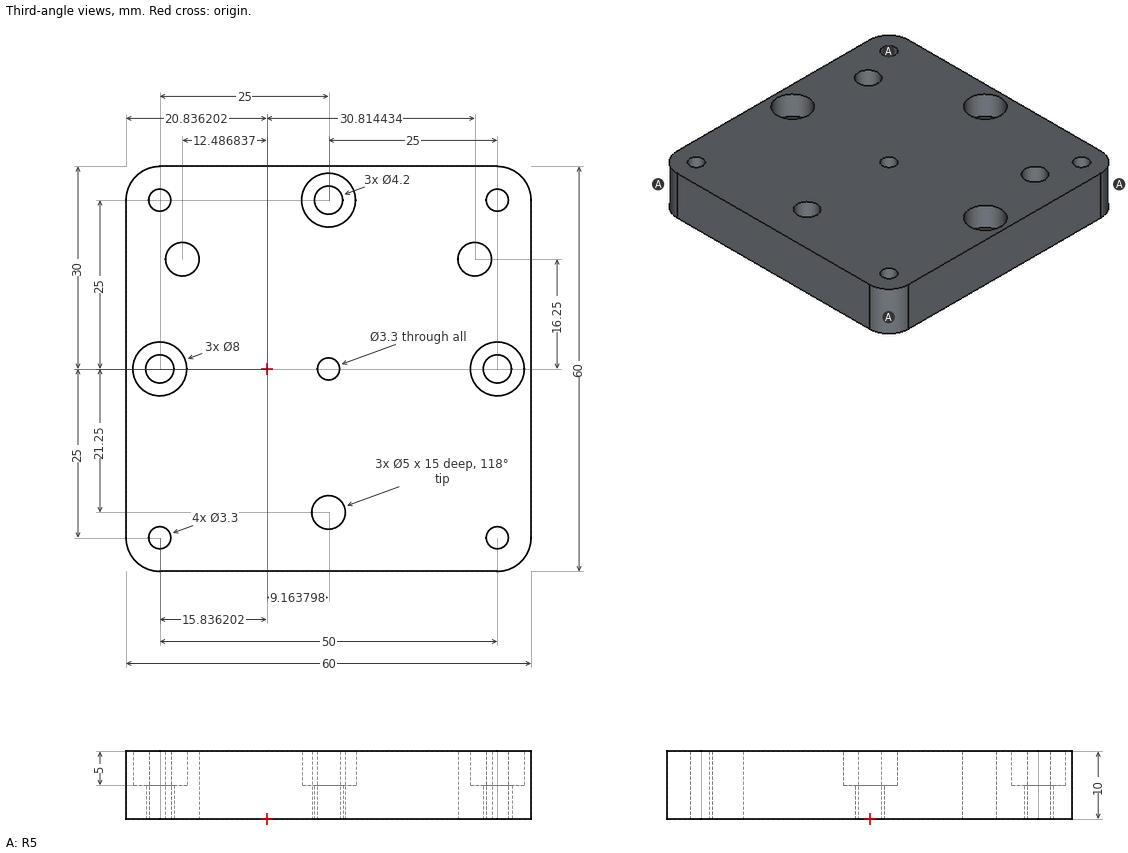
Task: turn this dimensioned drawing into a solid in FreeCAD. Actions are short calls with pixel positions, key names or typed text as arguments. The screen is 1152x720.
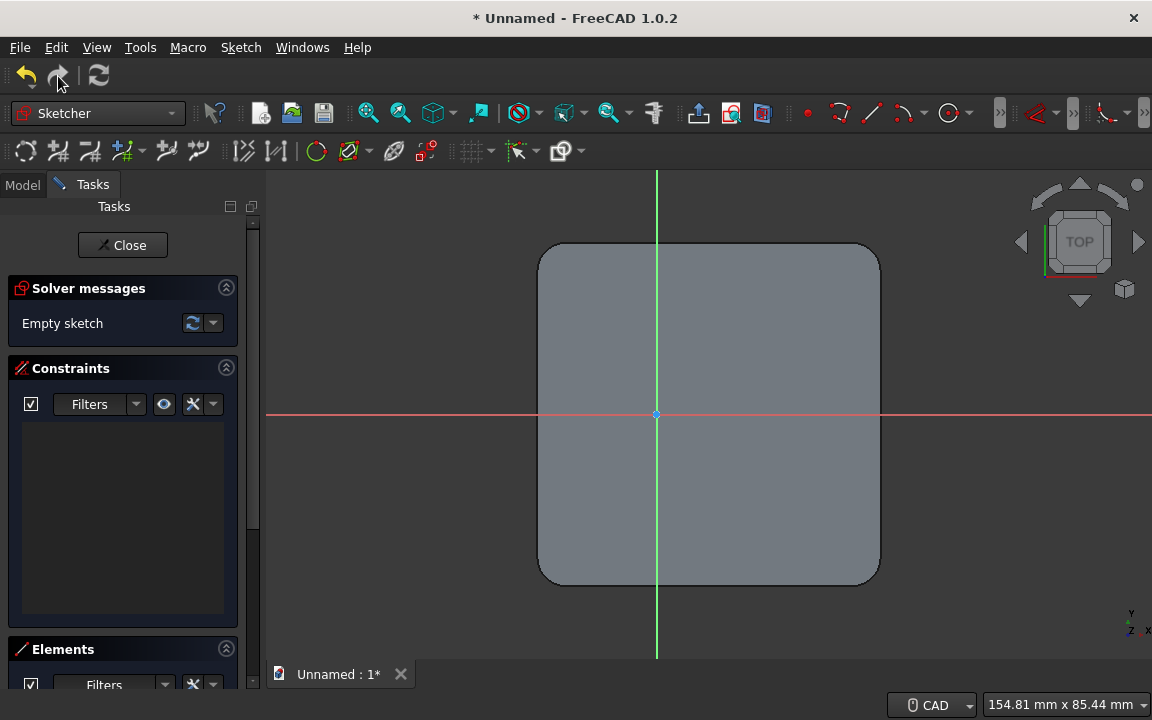
click(950, 114)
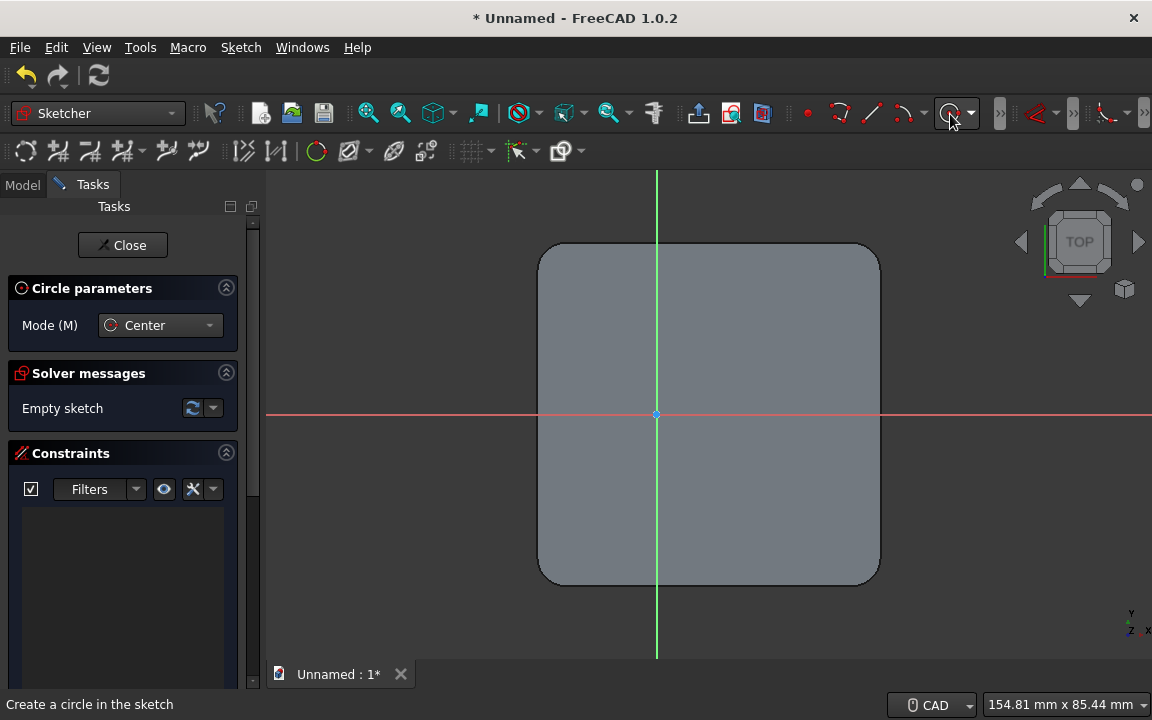
scroll(709, 536, up, 3)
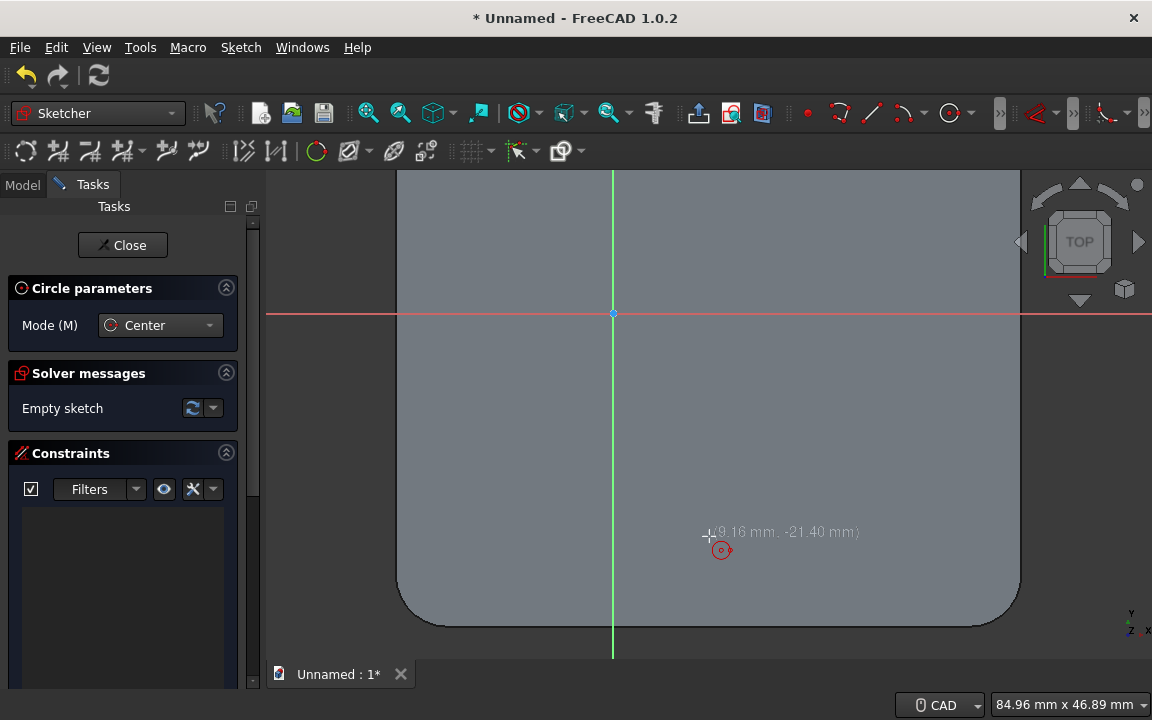
click(709, 536)
move(727, 517)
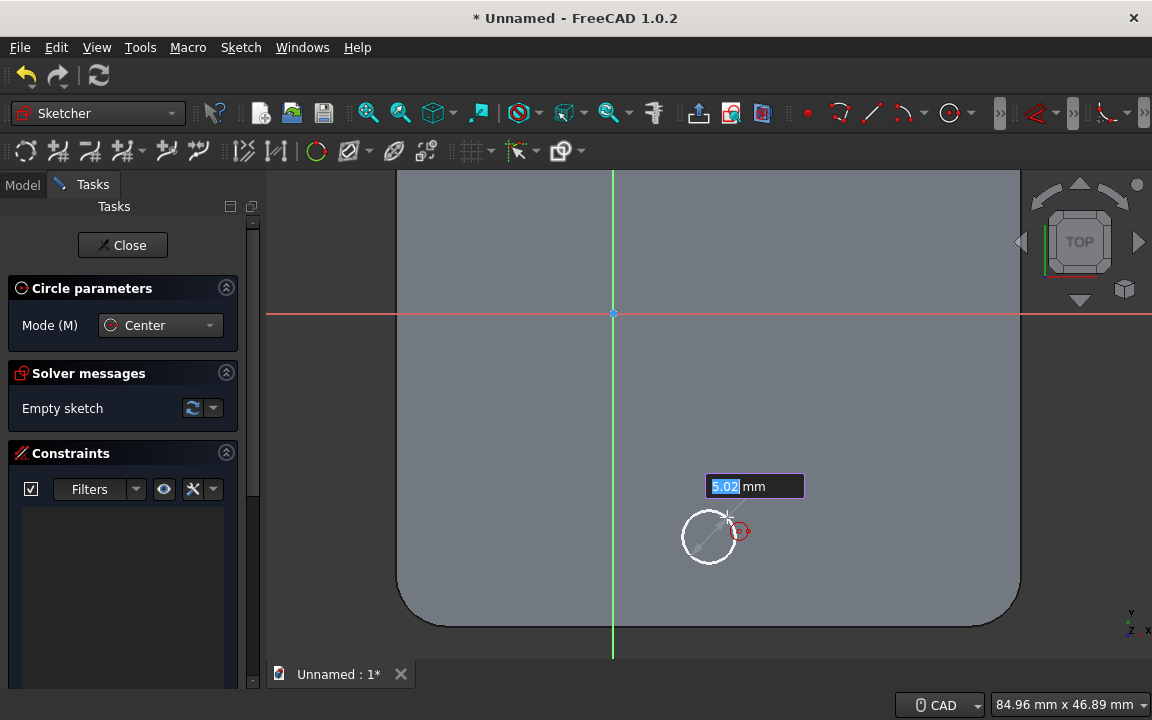
text(5)
key(Return)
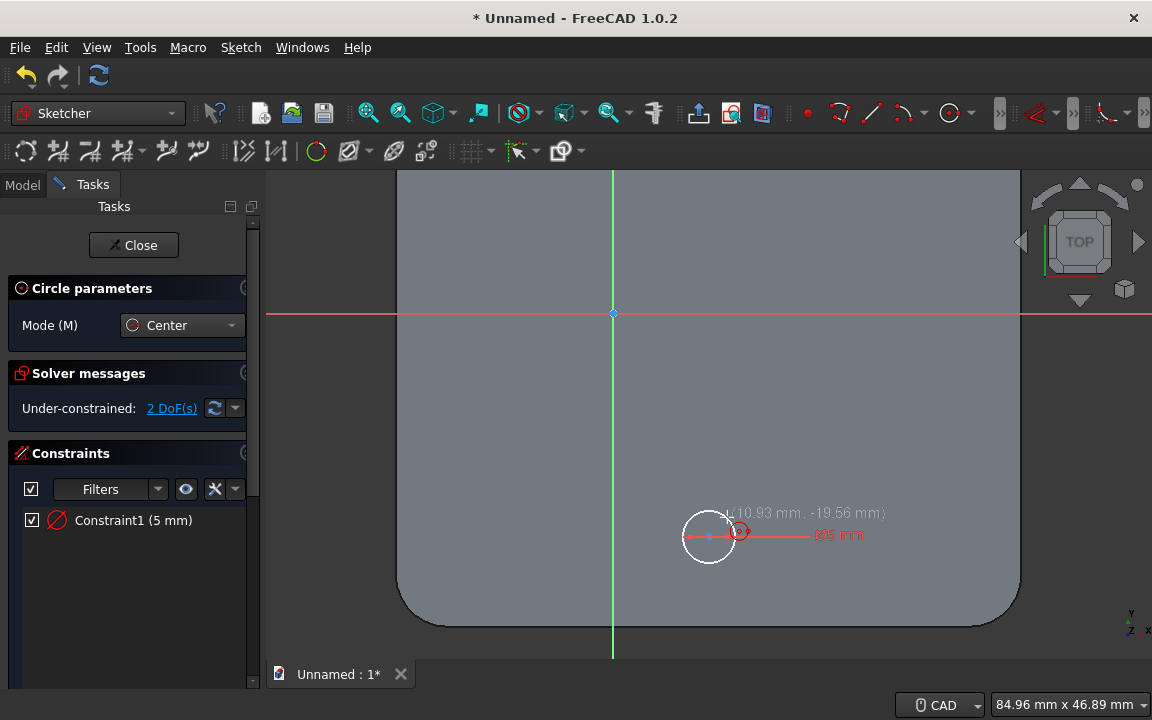
scroll(502, 566, down, 2)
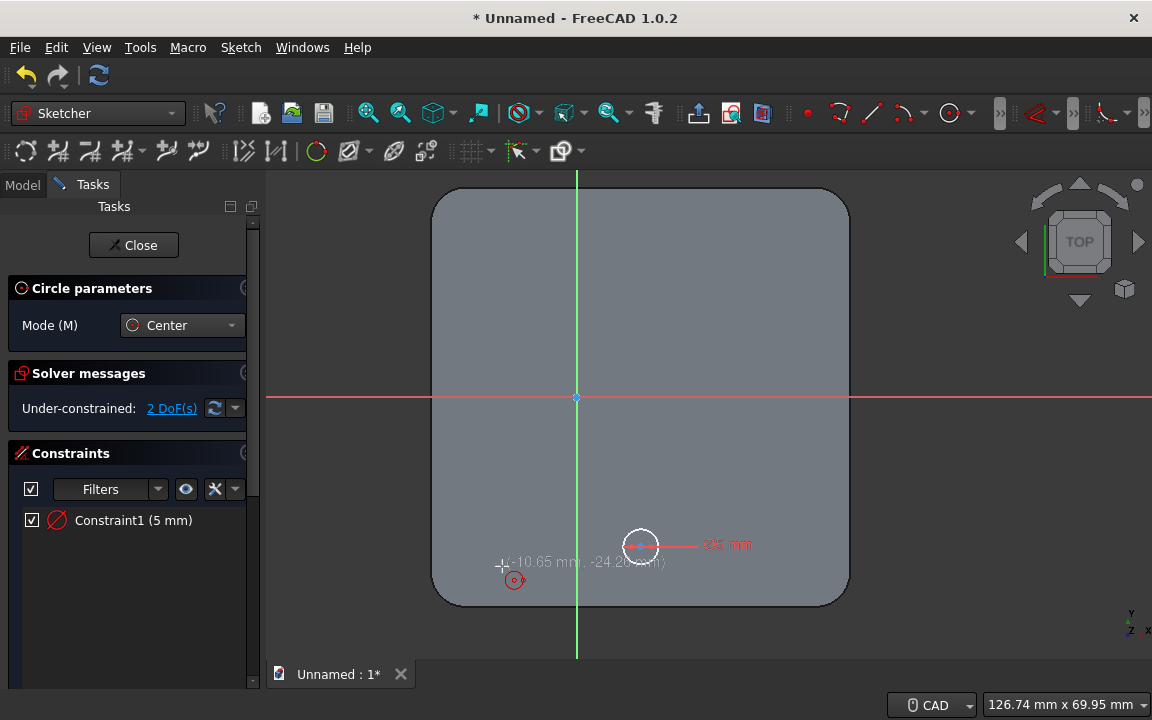
scroll(792, 284, up, 2)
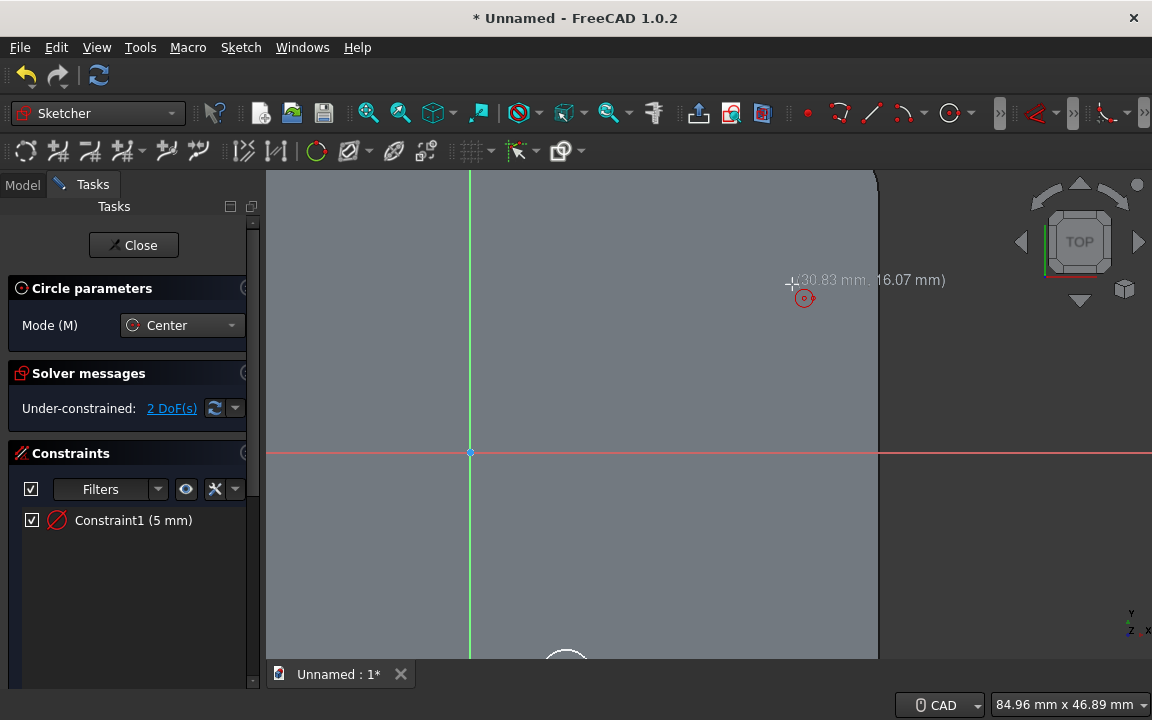
click(792, 284)
move(810, 265)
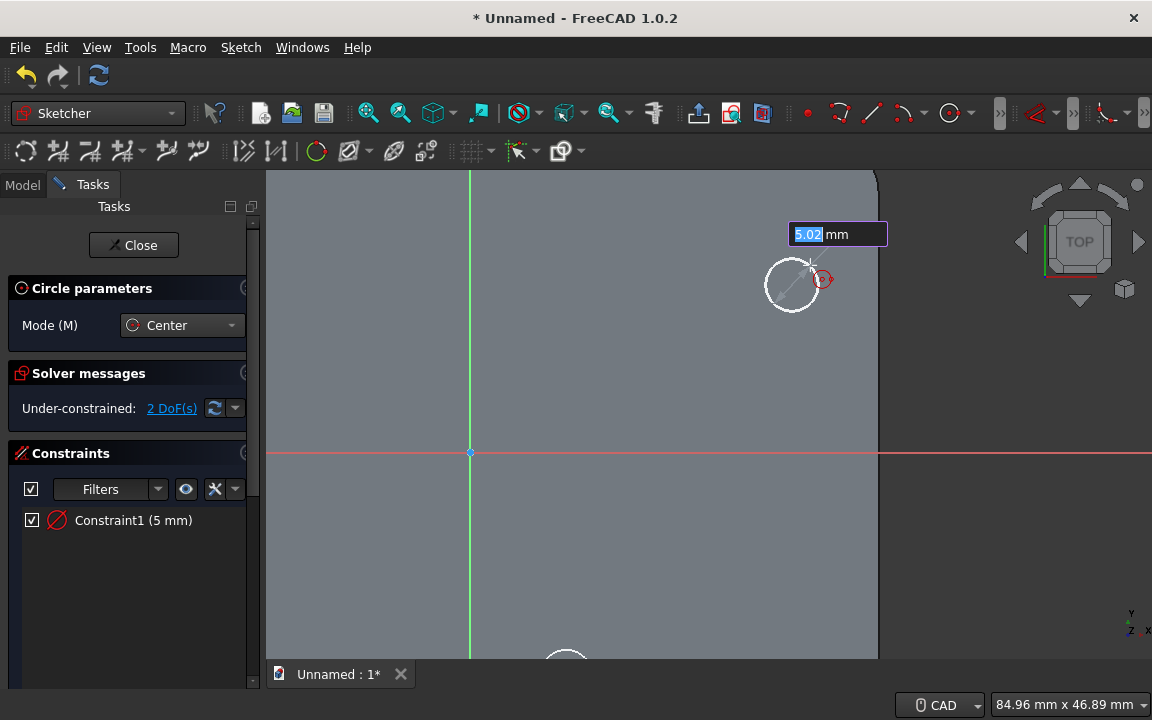
text(5)
key(Return)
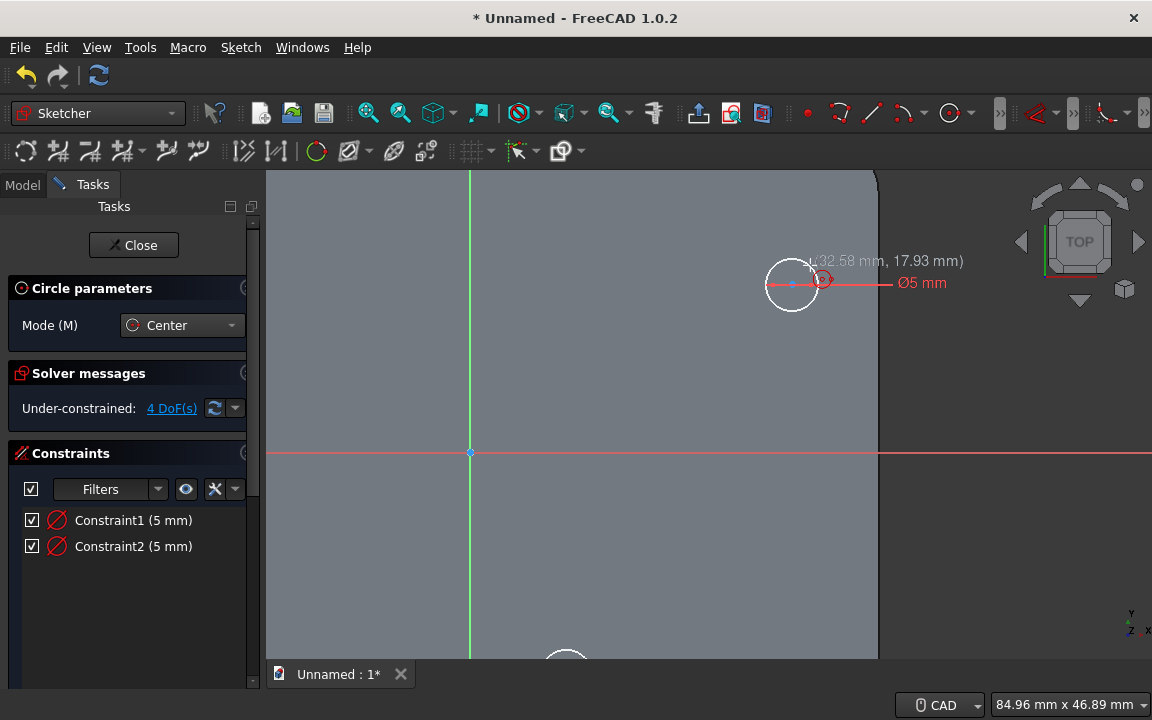
click(340, 284)
move(358, 265)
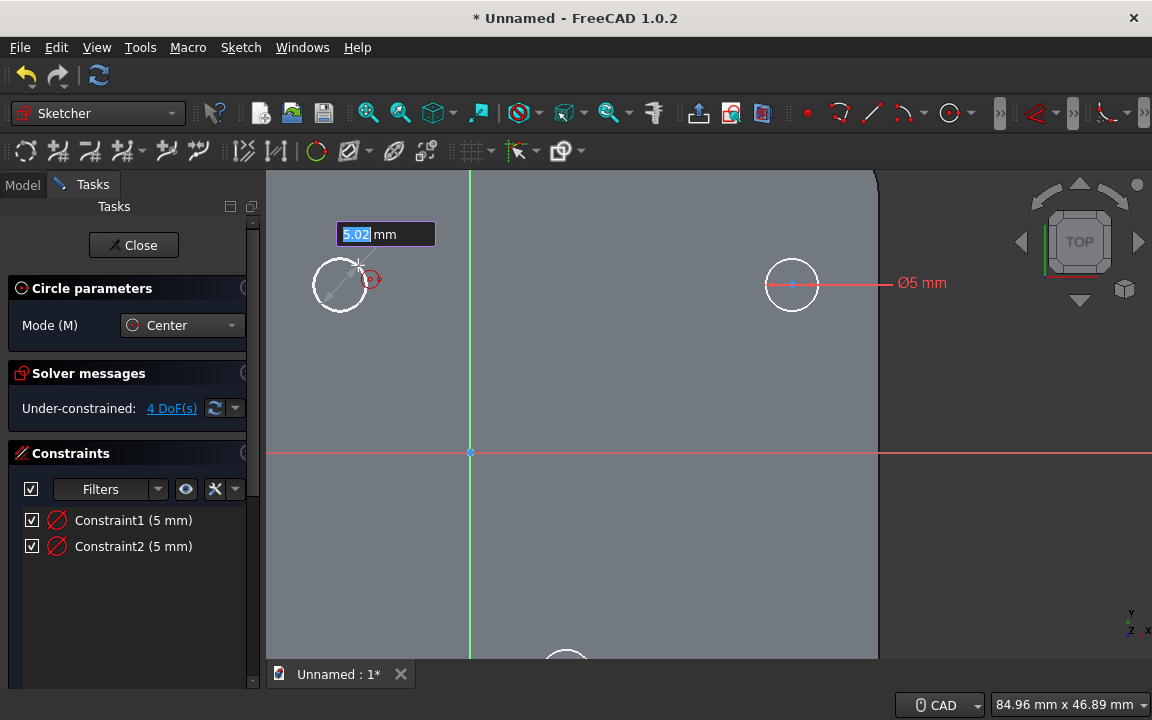
text(5)
key(Return)
key(Escape)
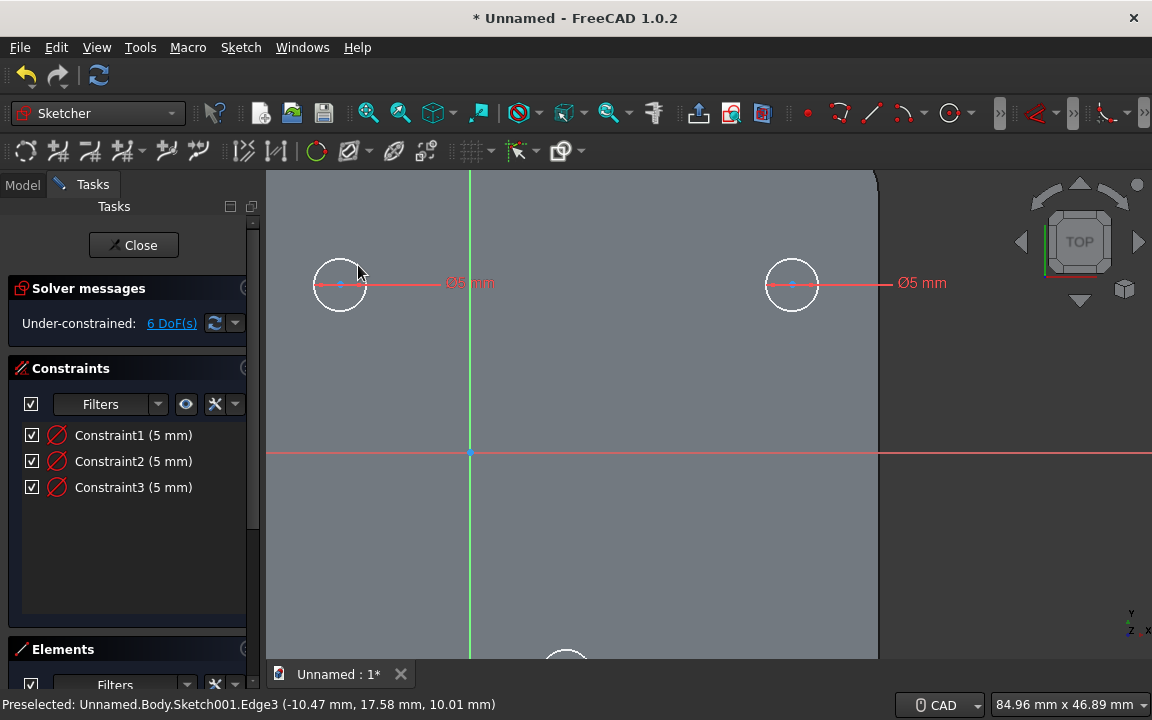
click(792, 285)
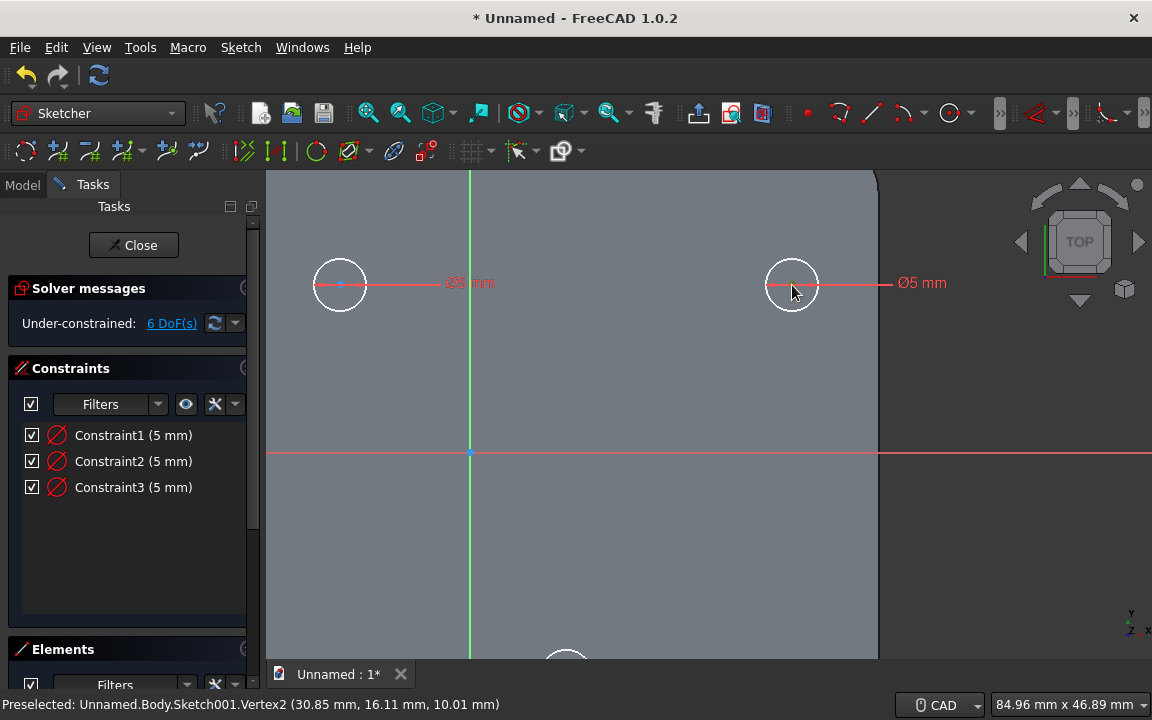
click(340, 285)